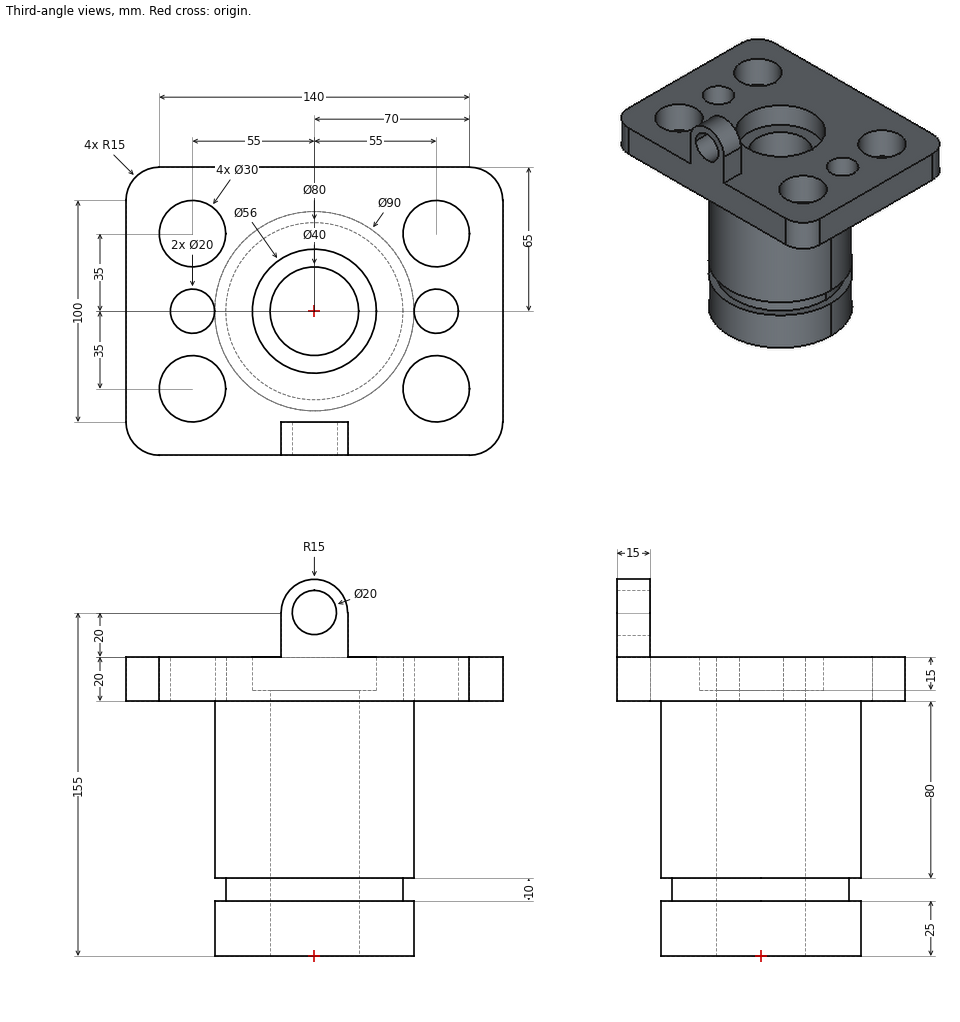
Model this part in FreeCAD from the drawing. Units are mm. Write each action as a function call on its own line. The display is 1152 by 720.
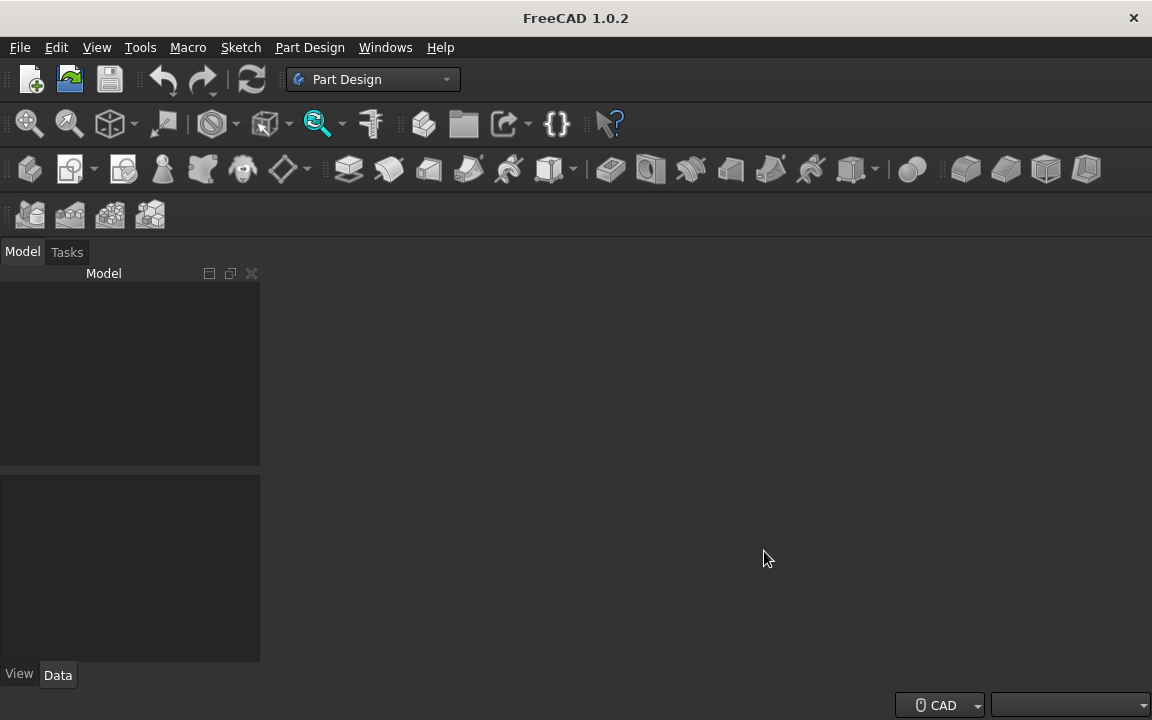
click(30, 80)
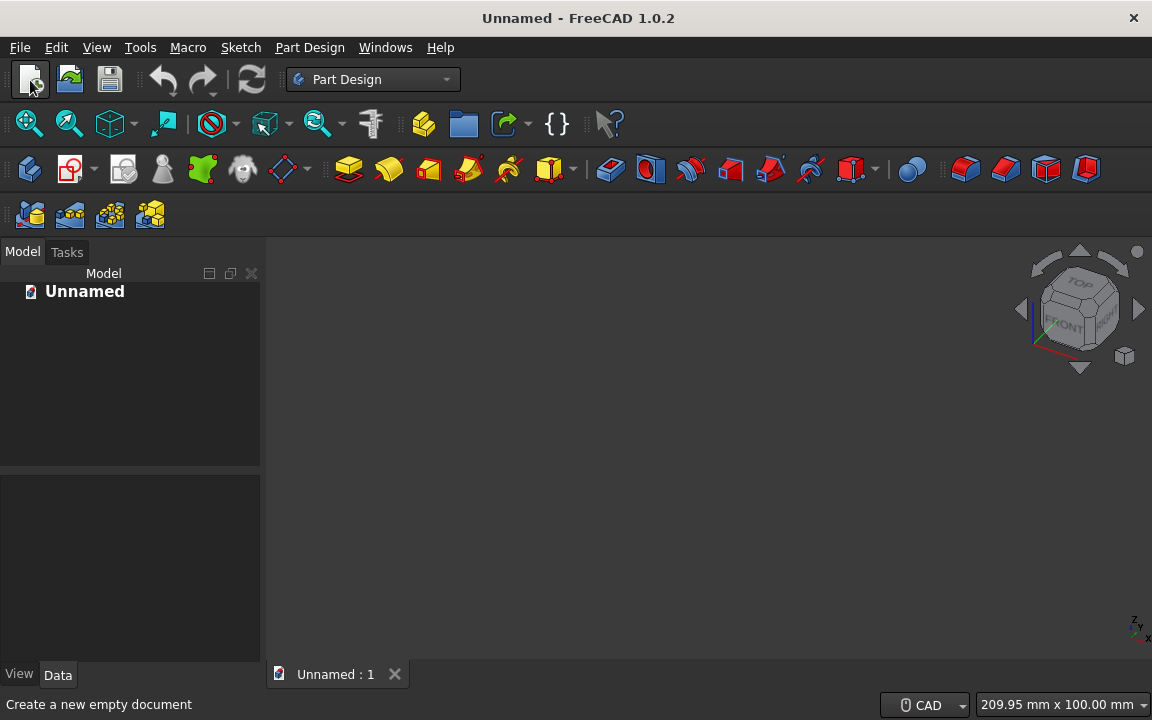
click(70, 170)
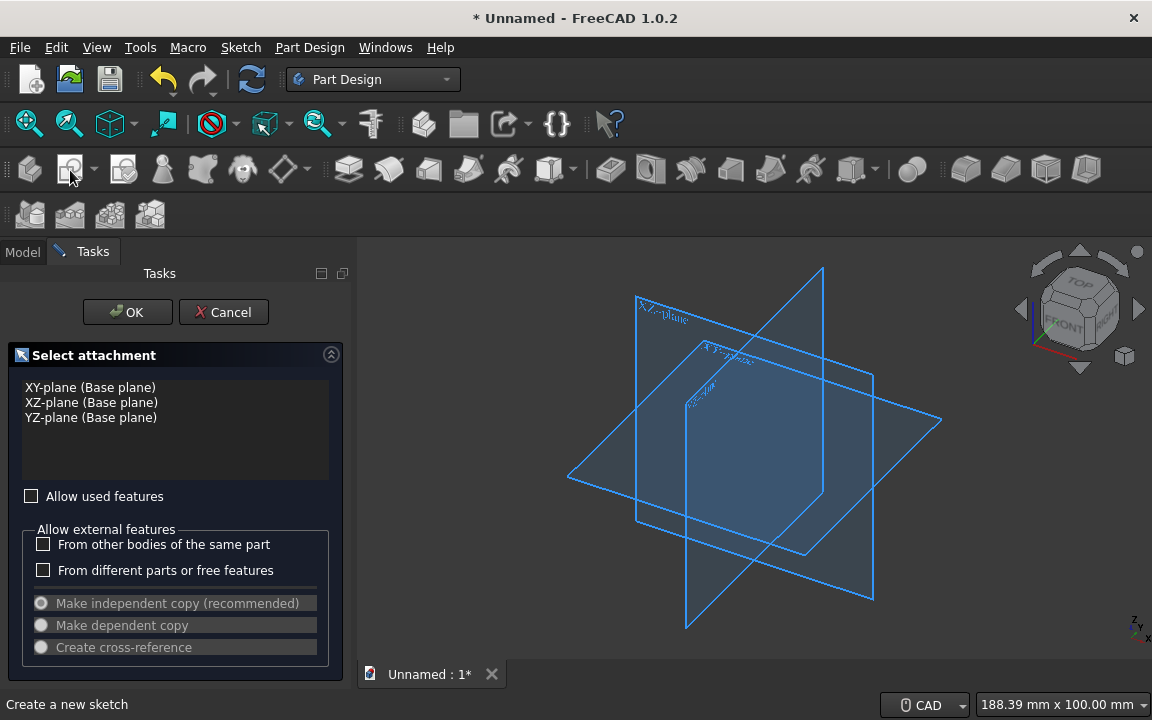
click(82, 388)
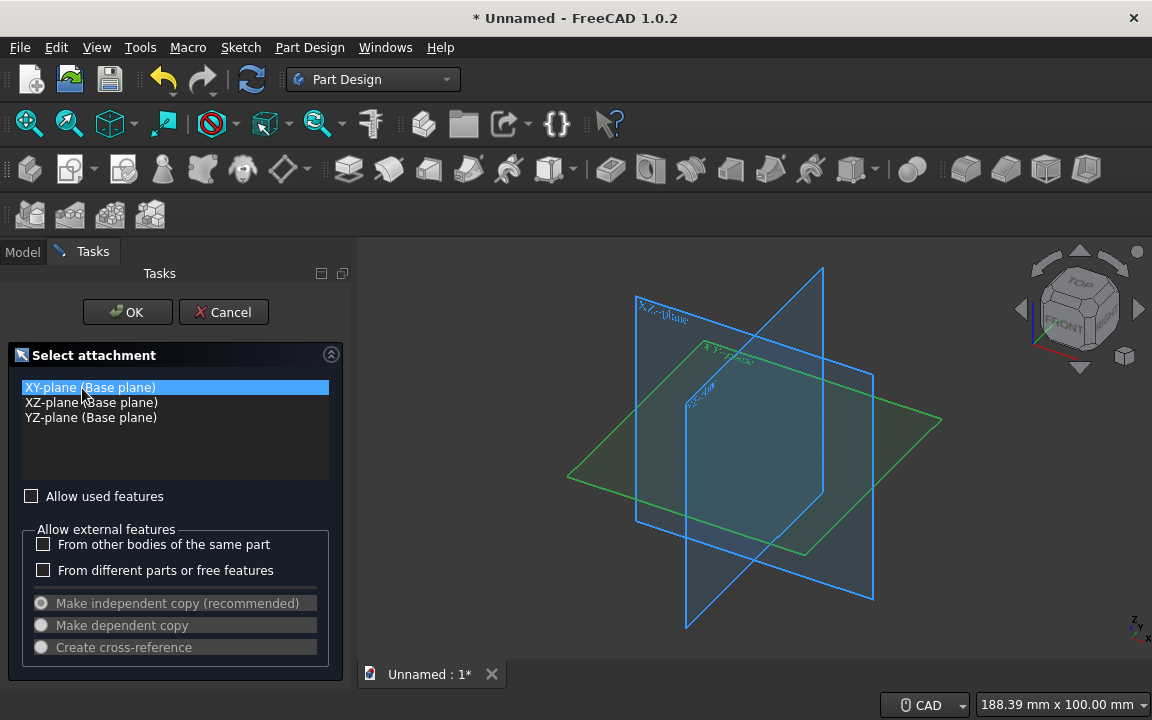
click(128, 312)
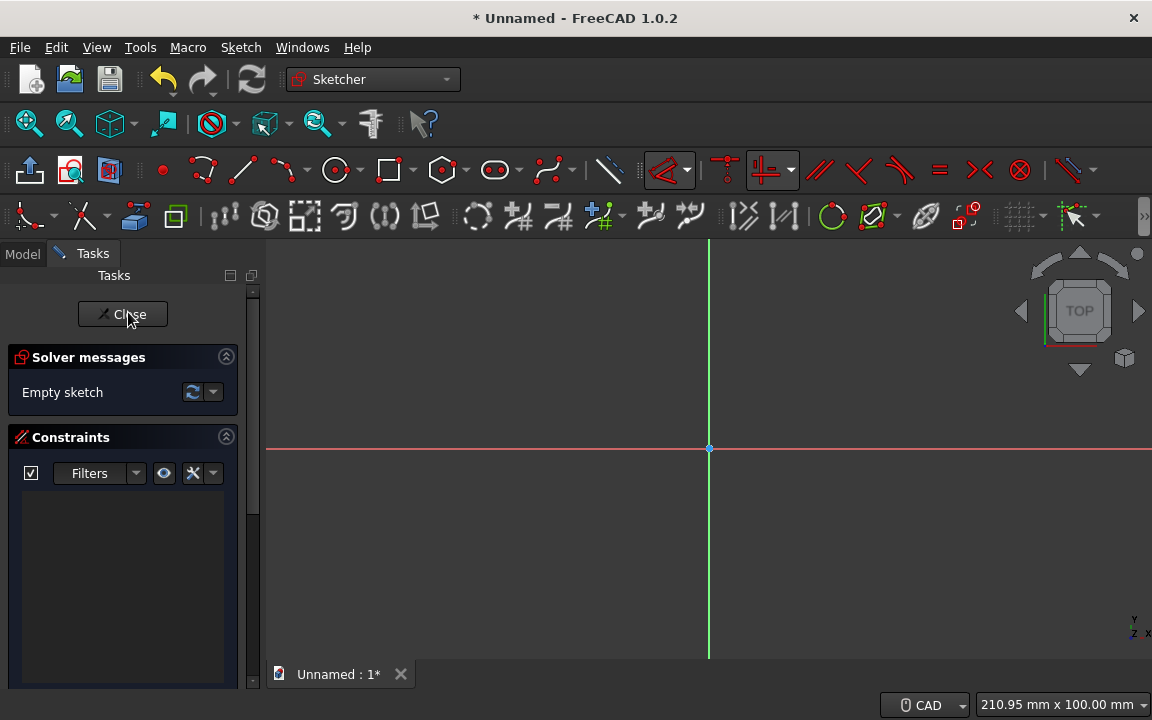
scroll(501, 449, down, 2)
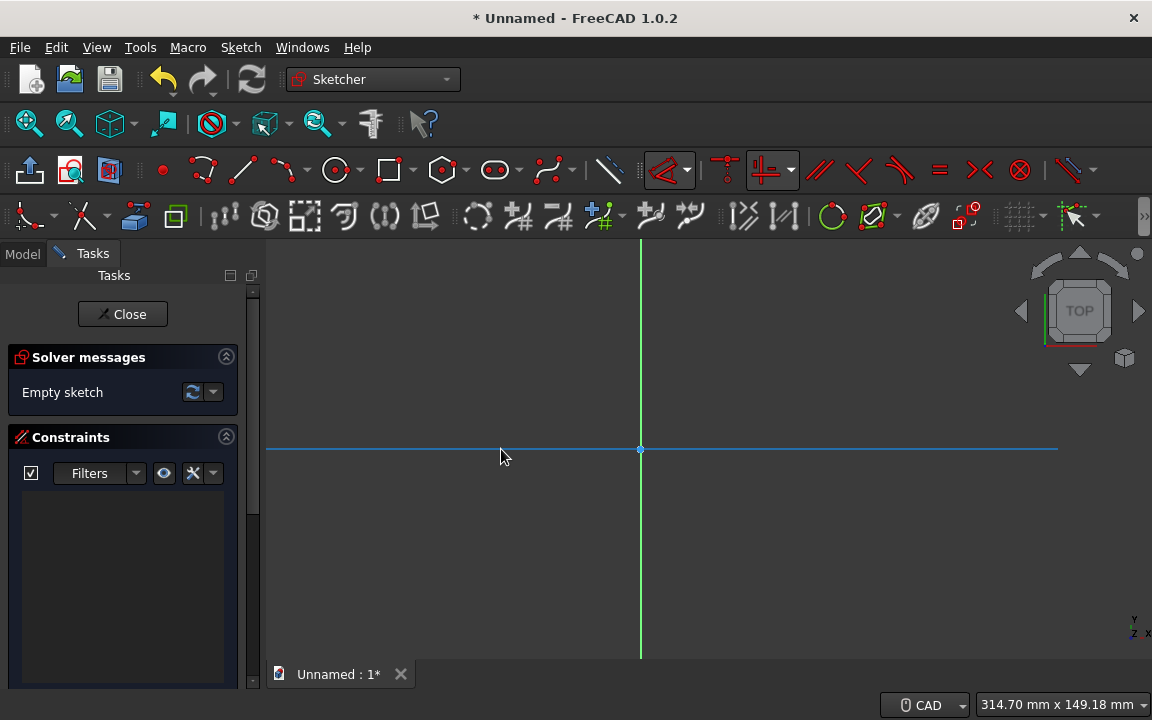
click(336, 170)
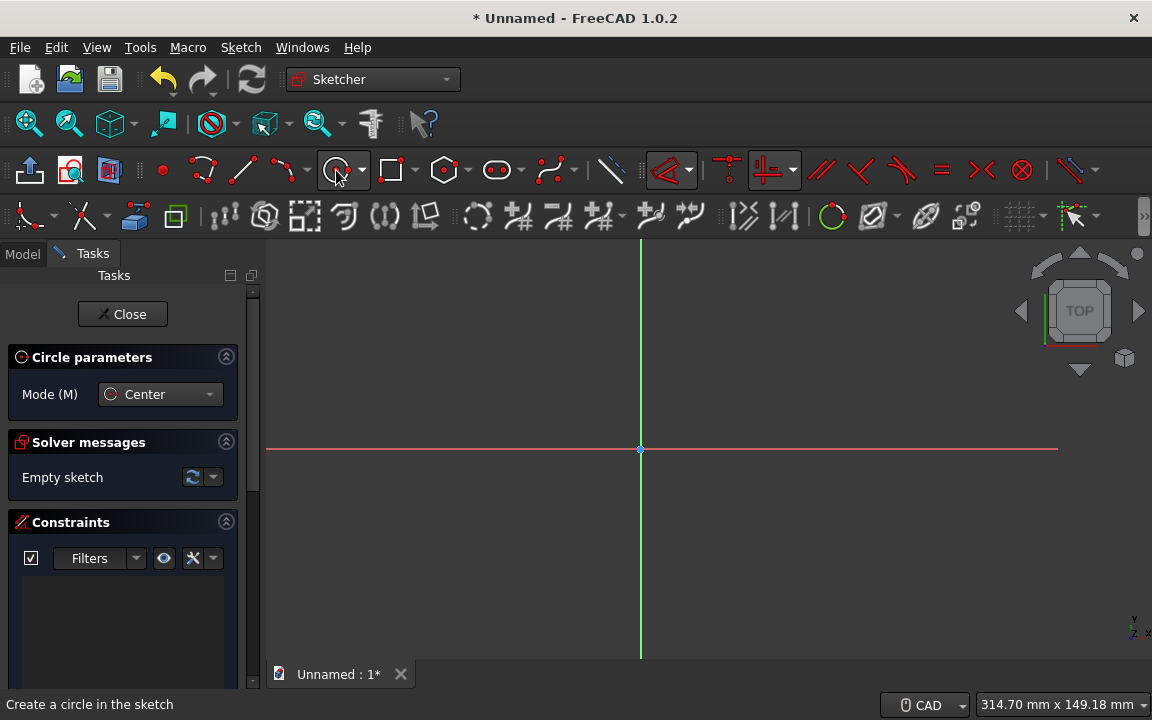
click(641, 449)
click(730, 360)
key(Escape)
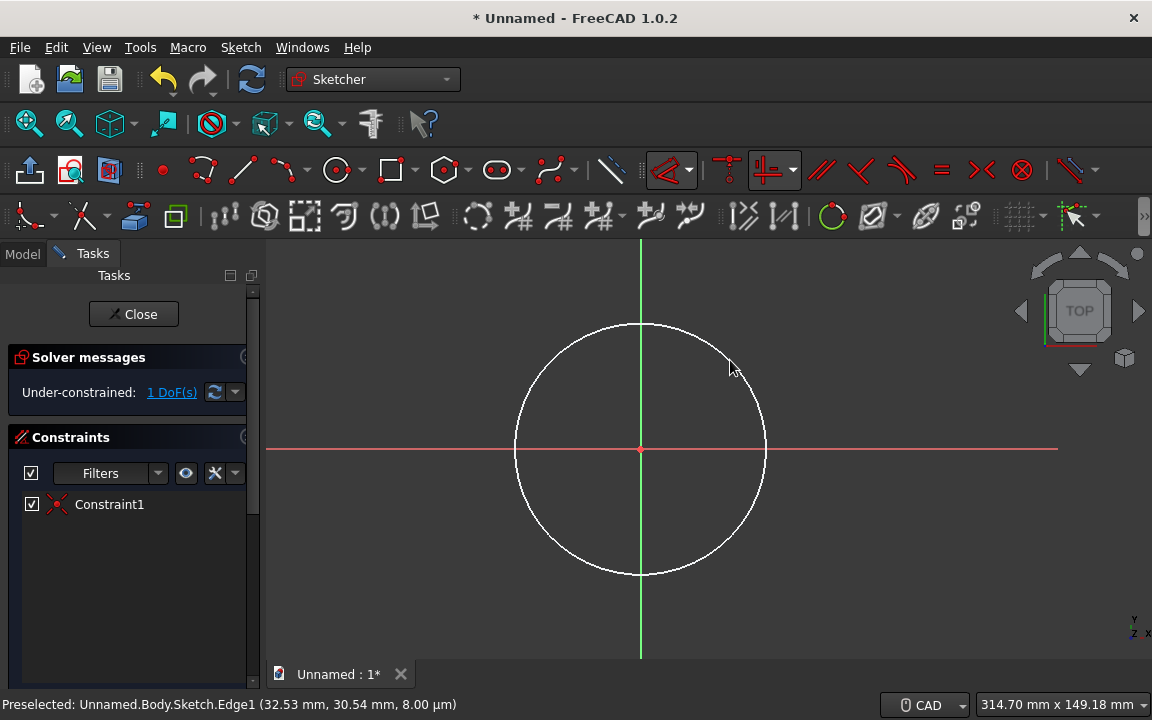
click(666, 170)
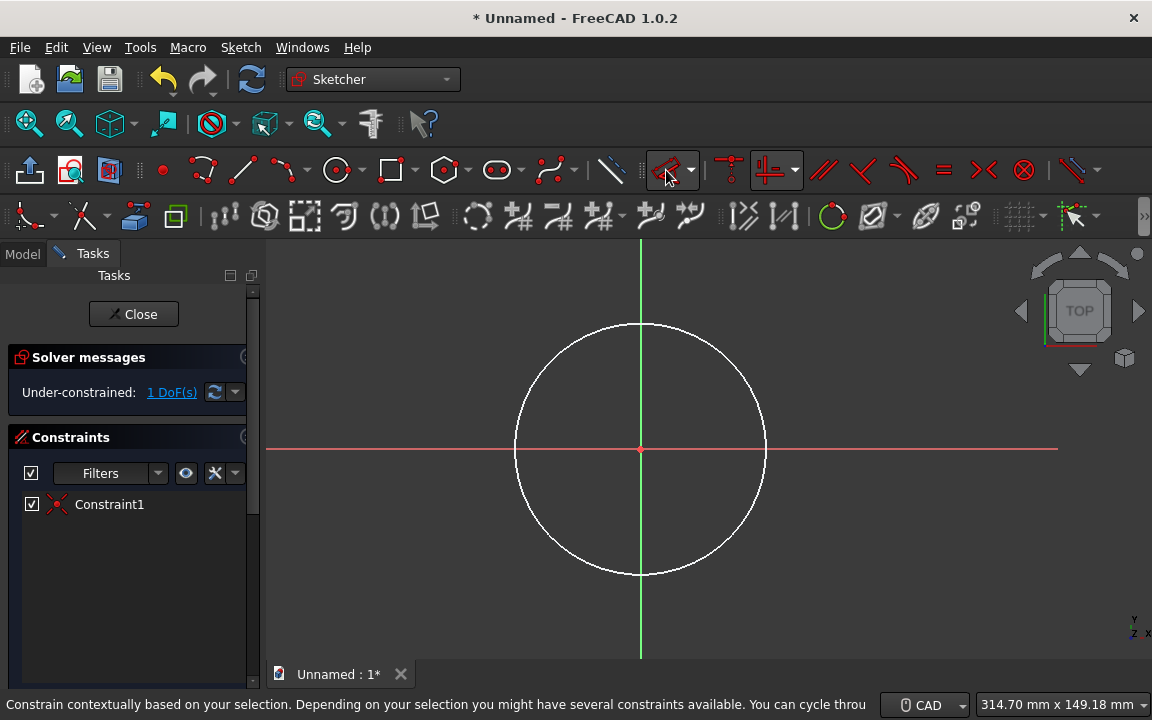
click(729, 360)
click(752, 337)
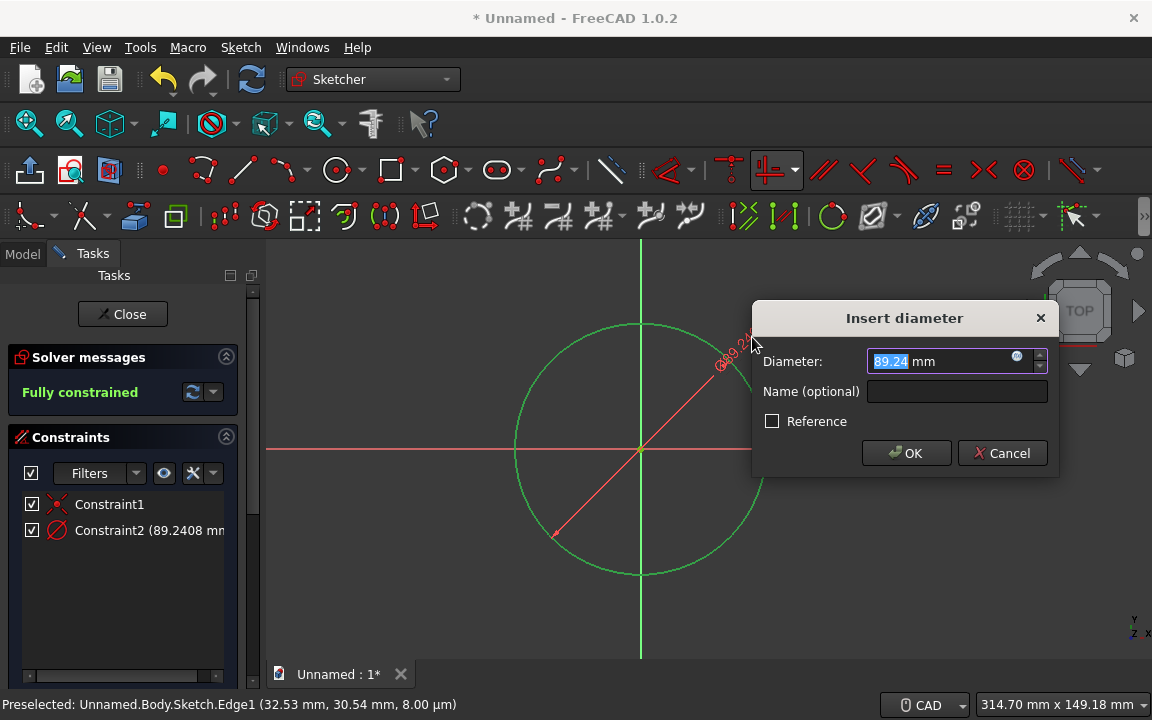
text(90)
key(Return)
key(Escape)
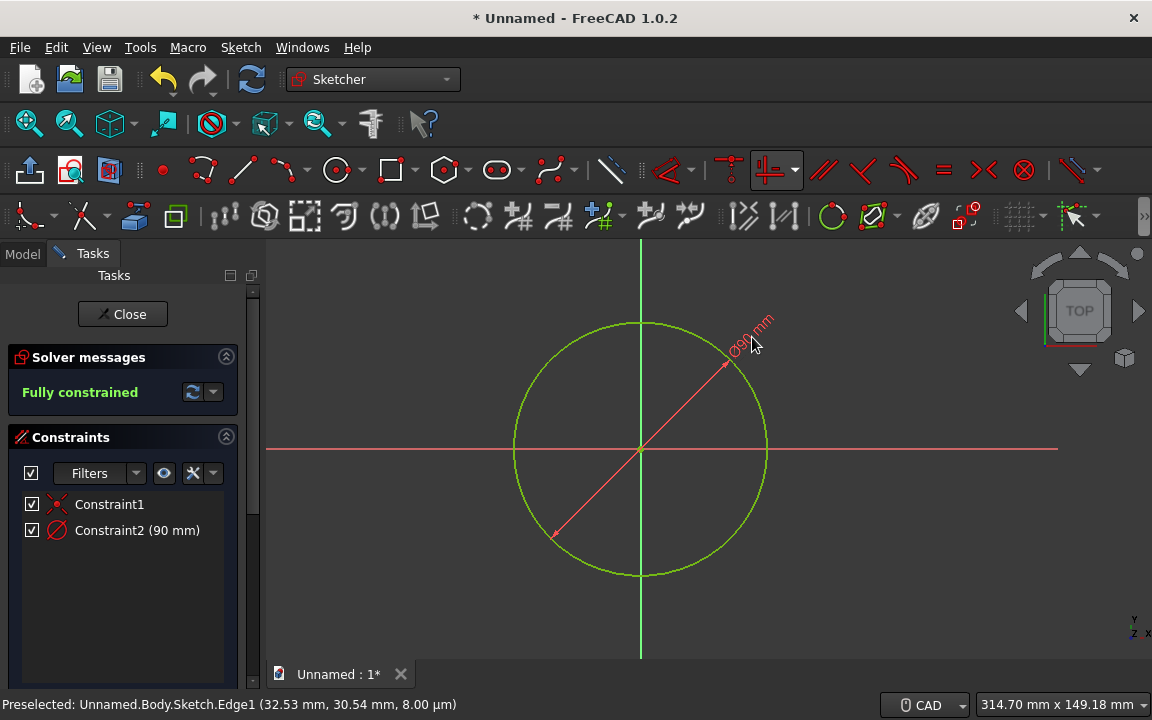
click(123, 314)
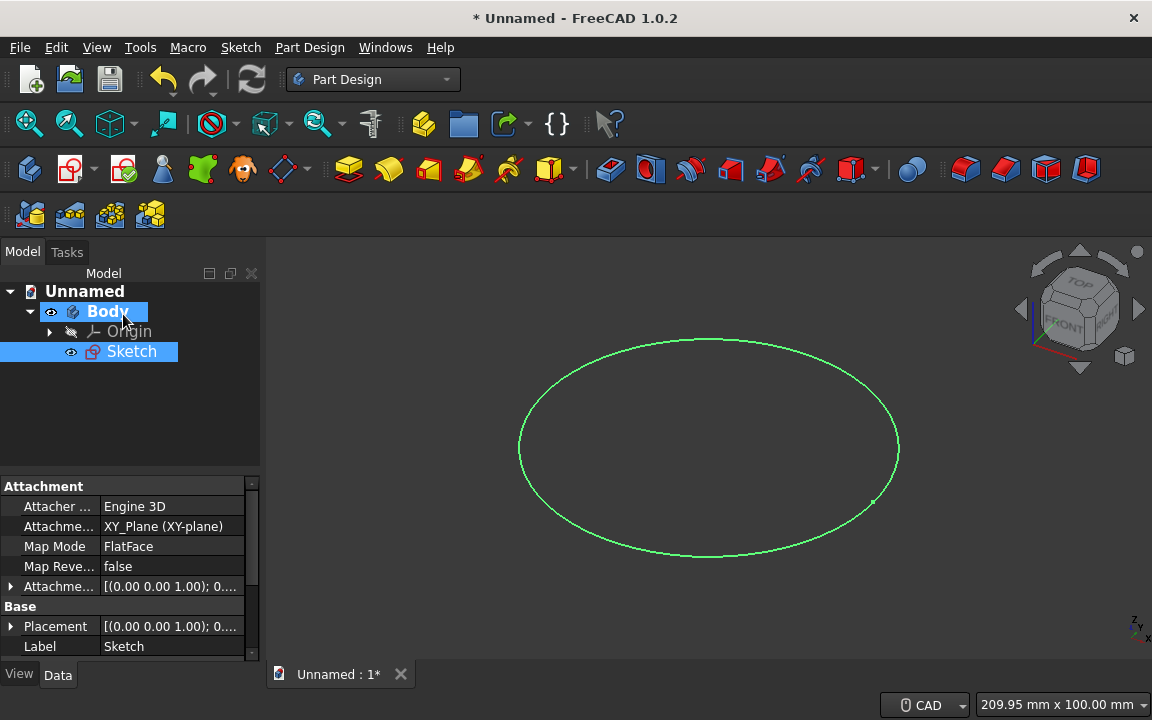
click(350, 170)